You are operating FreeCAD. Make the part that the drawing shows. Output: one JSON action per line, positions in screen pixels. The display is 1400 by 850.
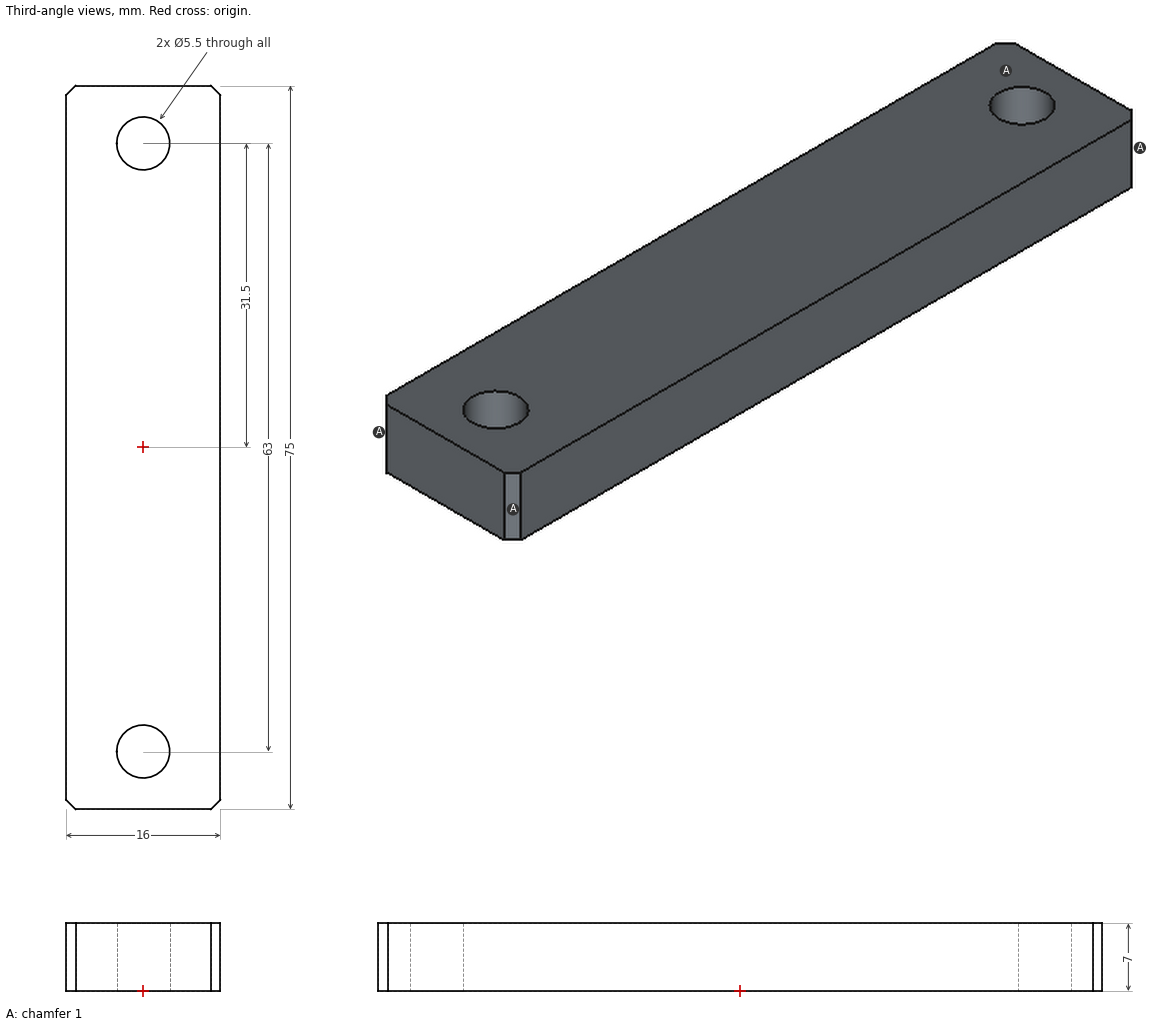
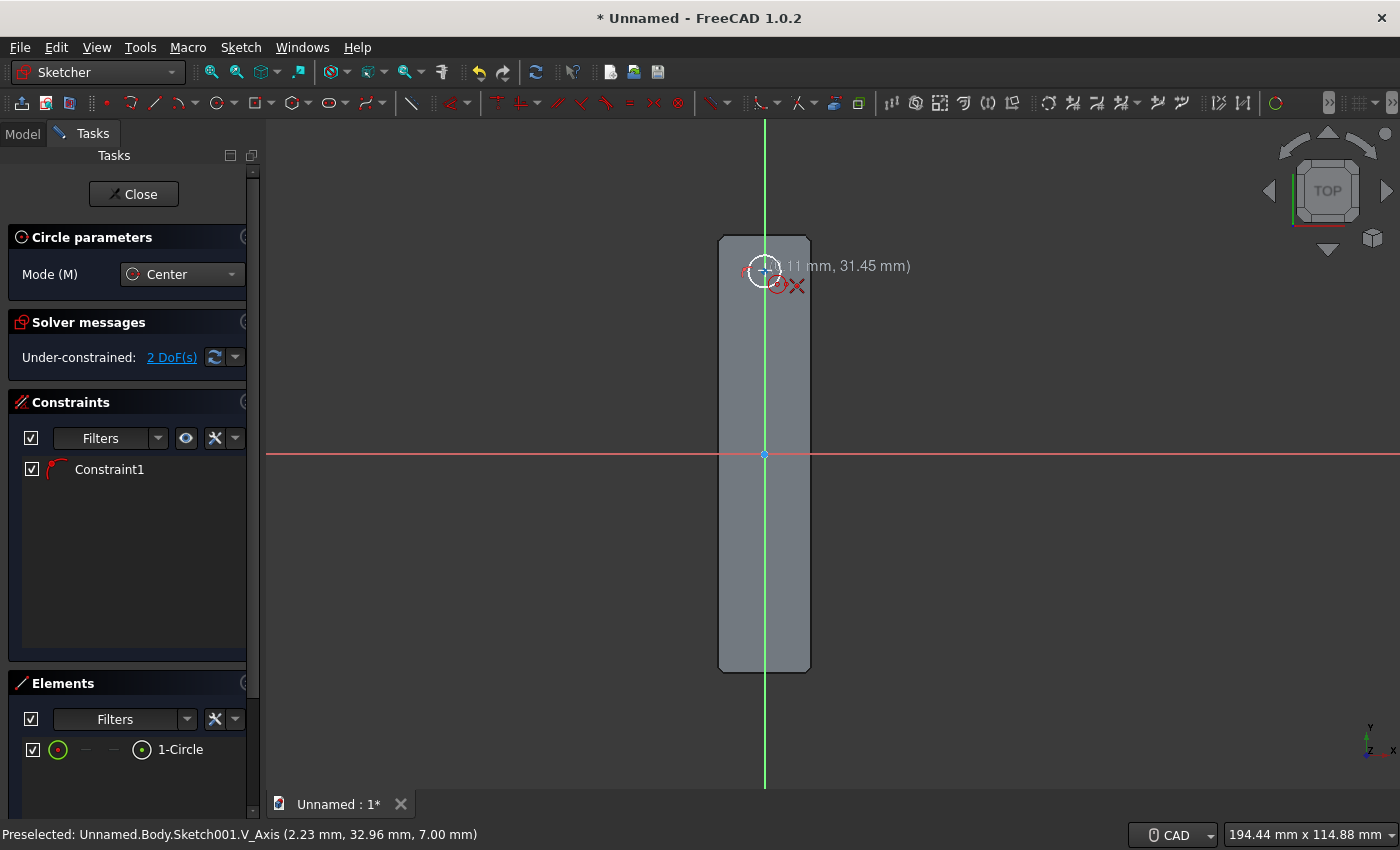
{"action": "scroll", "coordinate": [765, 638], "scroll_direction": "up", "scroll_amount": 2}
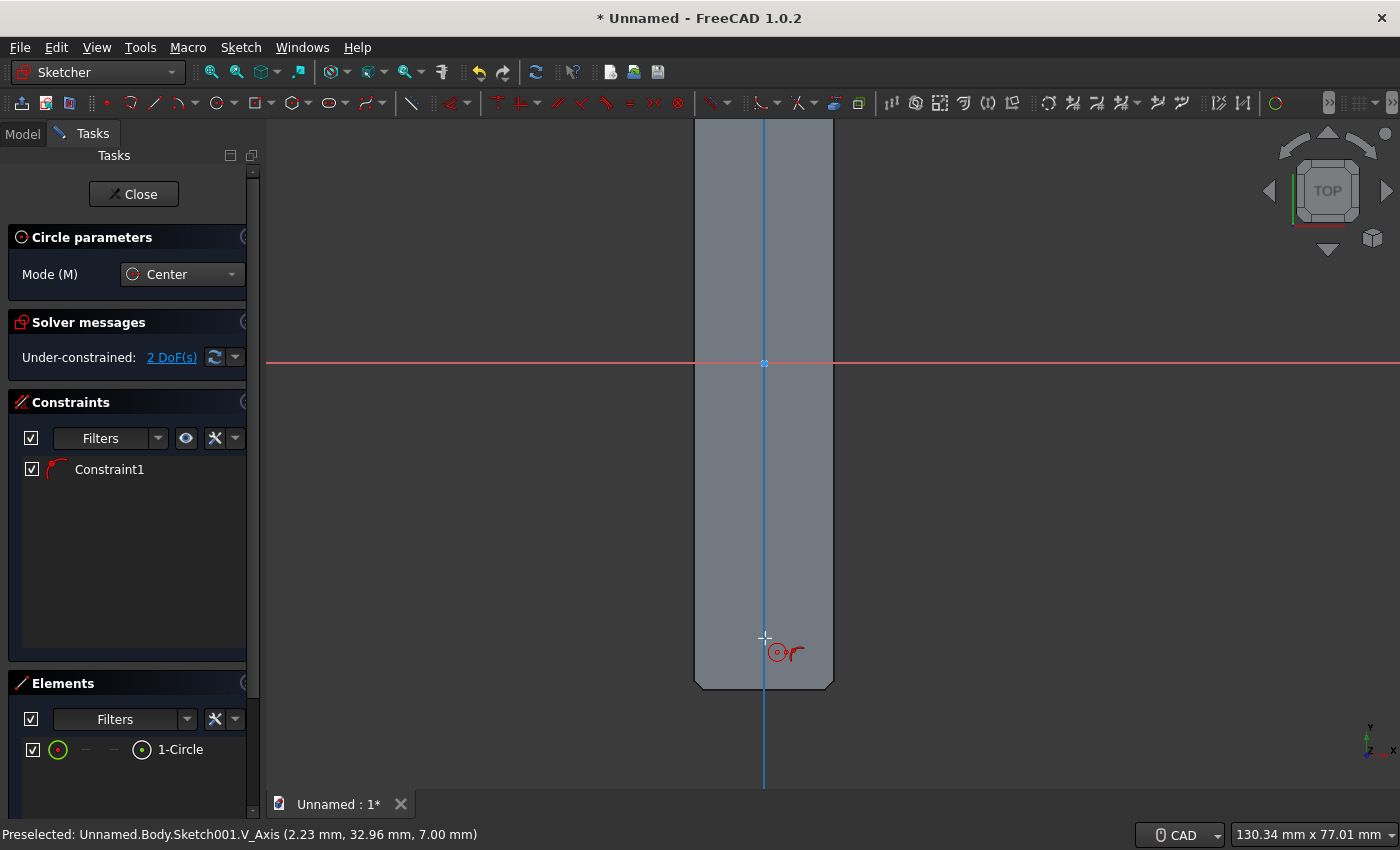
{"action": "left_click", "coordinate": [764, 637]}
{"action": "left_click", "coordinate": [781, 621]}
{"action": "key", "text": "Escape"}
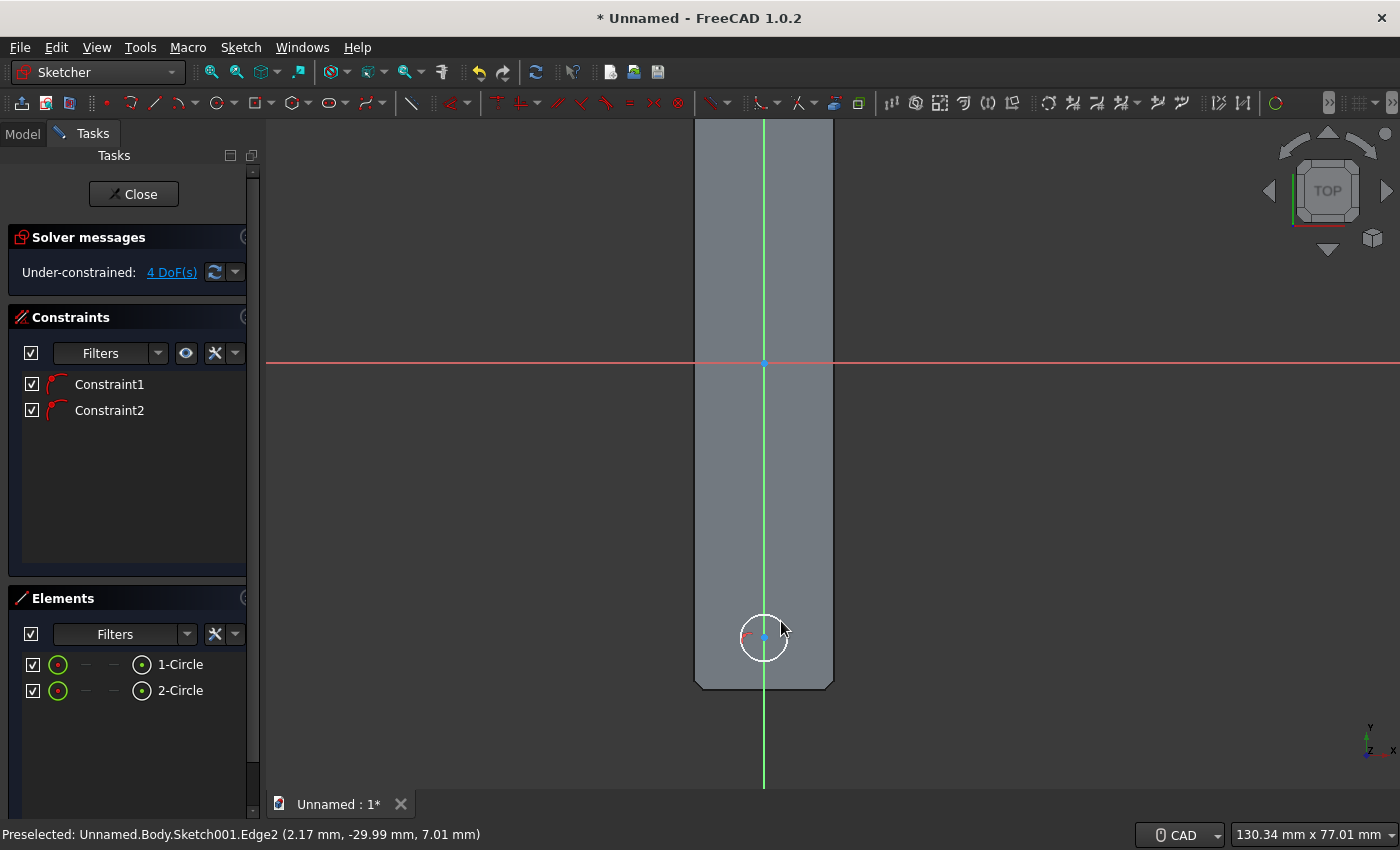
{"action": "scroll", "coordinate": [765, 638], "scroll_direction": "down", "scroll_amount": 2}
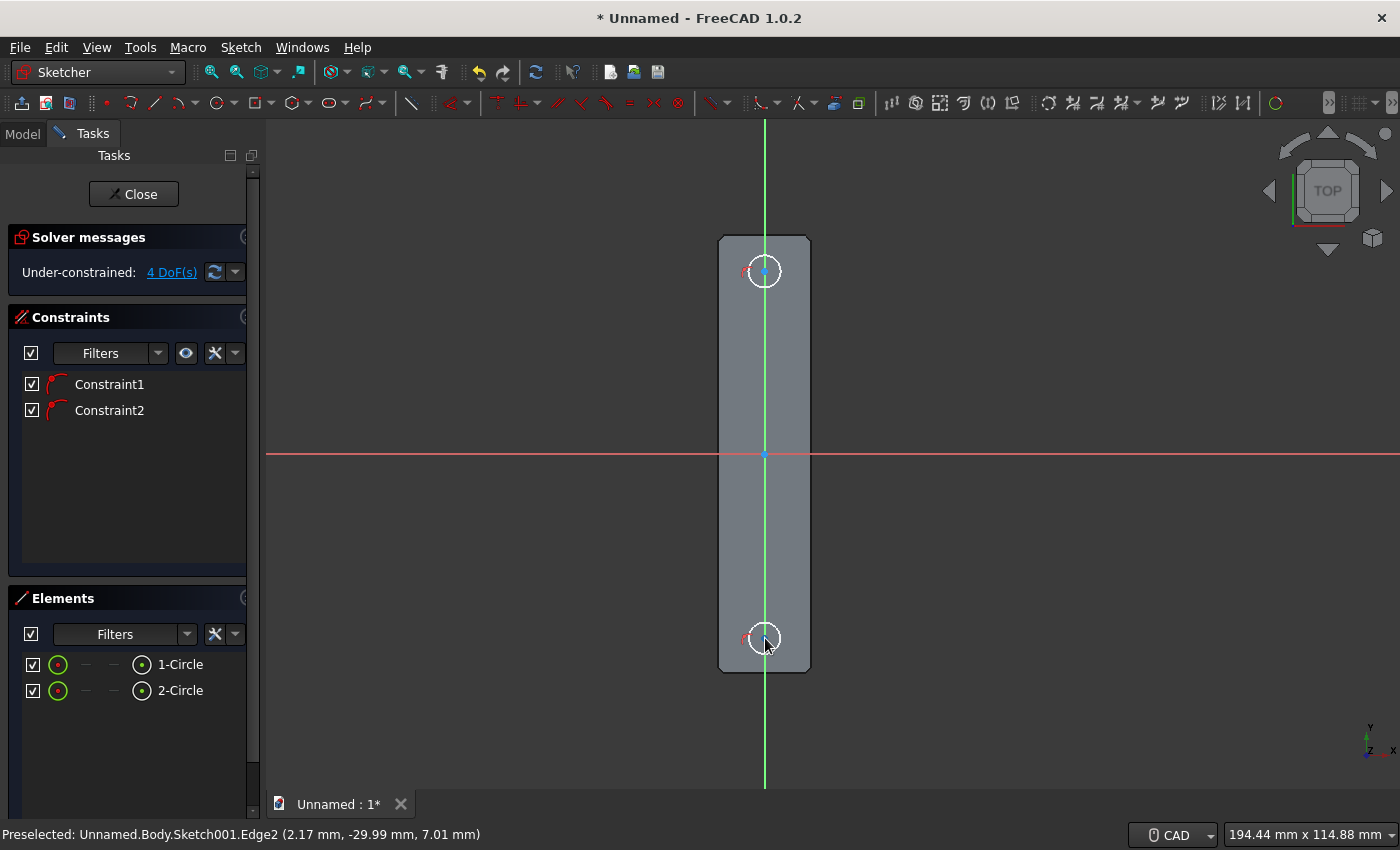
{"action": "left_click", "coordinate": [776, 260]}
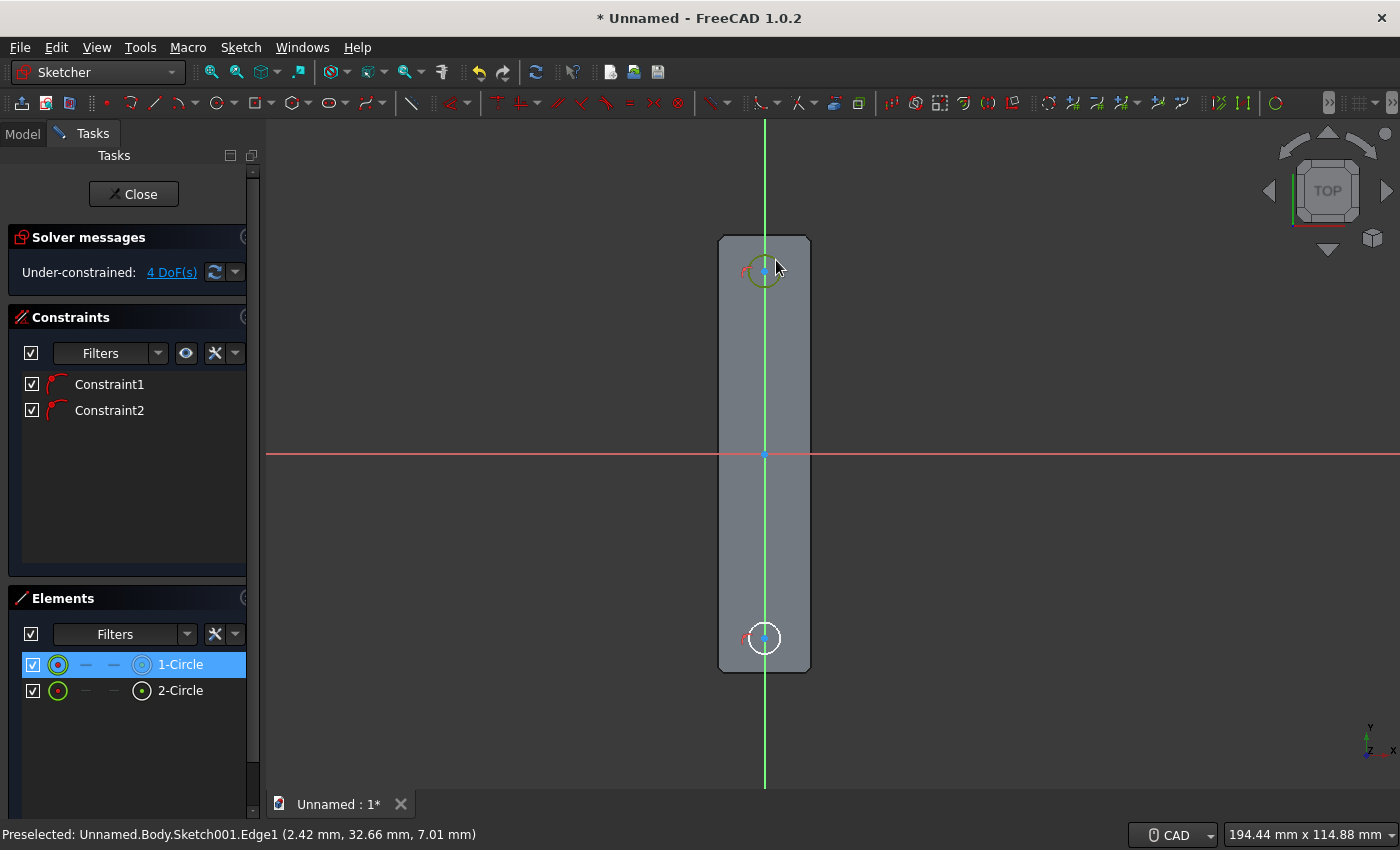
{"action": "scroll", "coordinate": [776, 627], "scroll_direction": "up", "scroll_amount": 2}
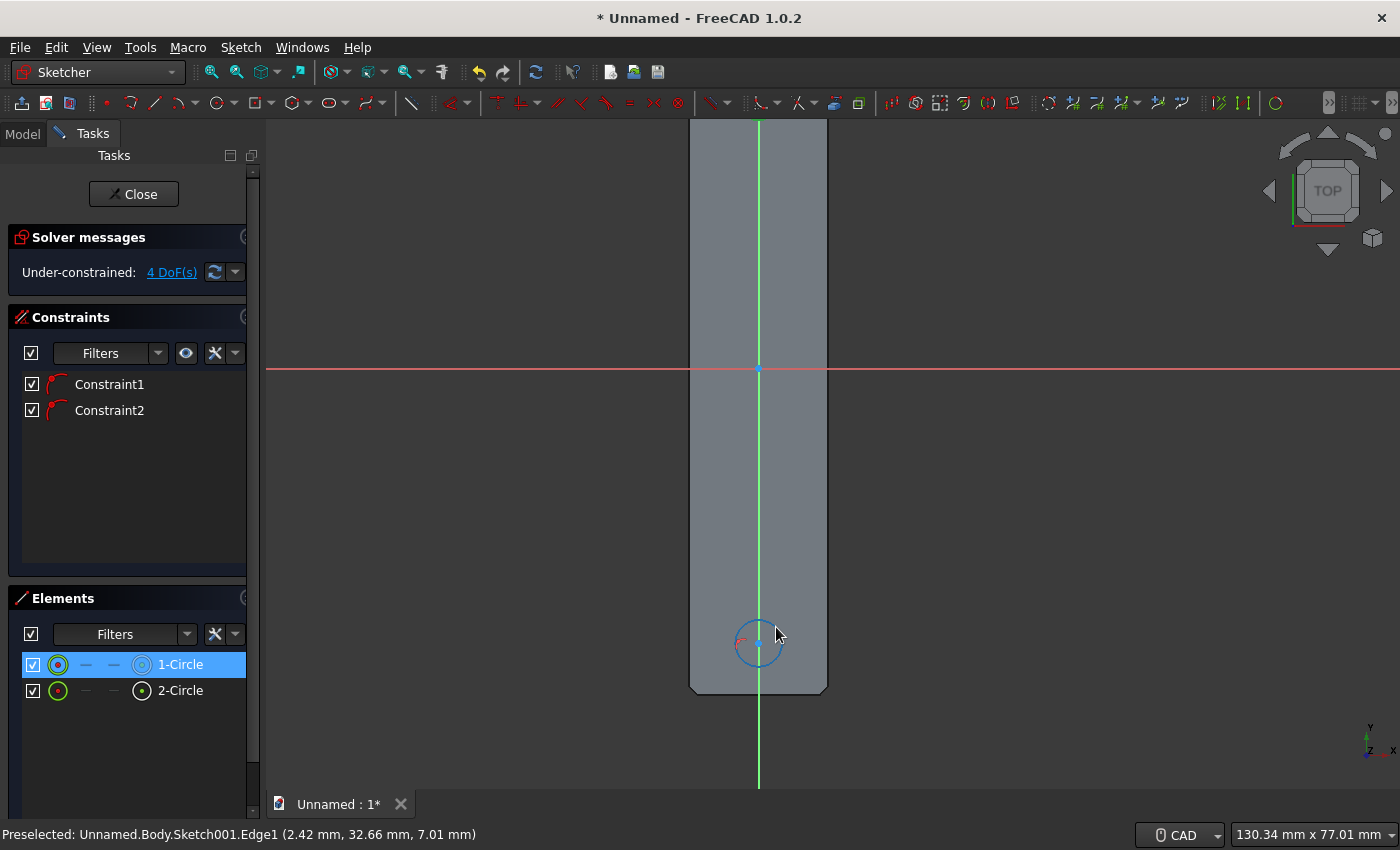
{"action": "left_click", "coordinate": [775, 627]}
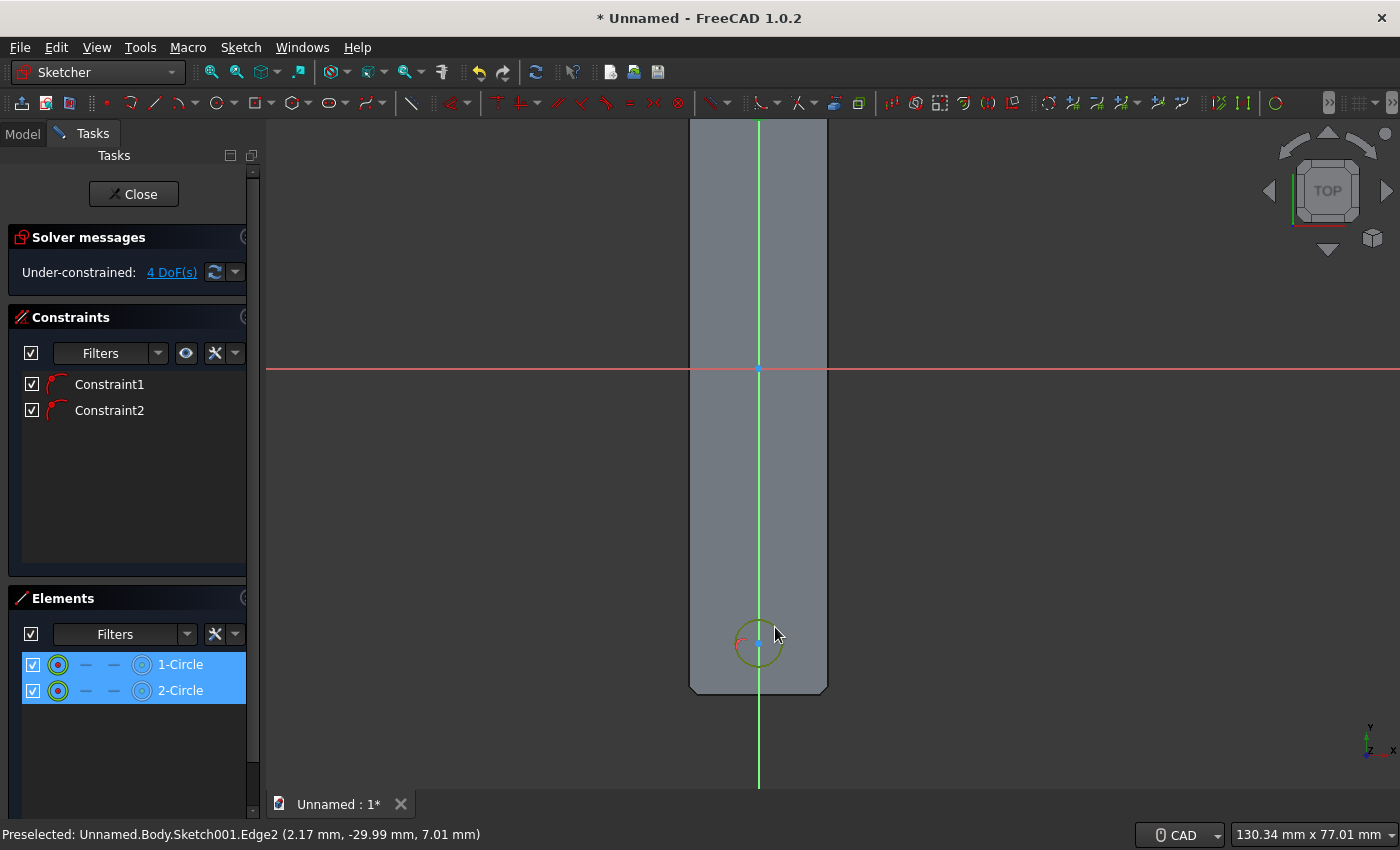
{"action": "left_click", "coordinate": [630, 104]}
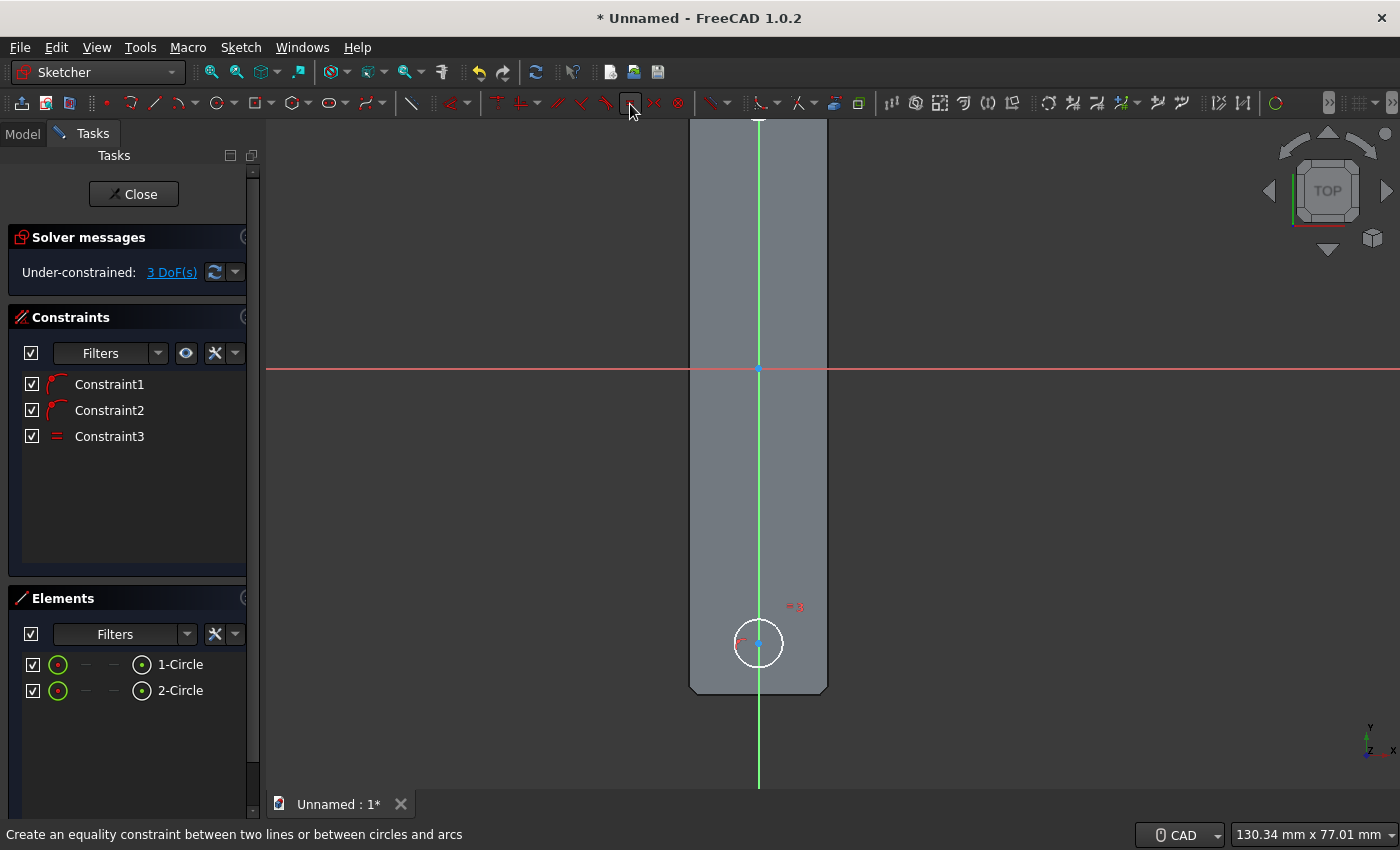
{"action": "left_click", "coordinate": [450, 104]}